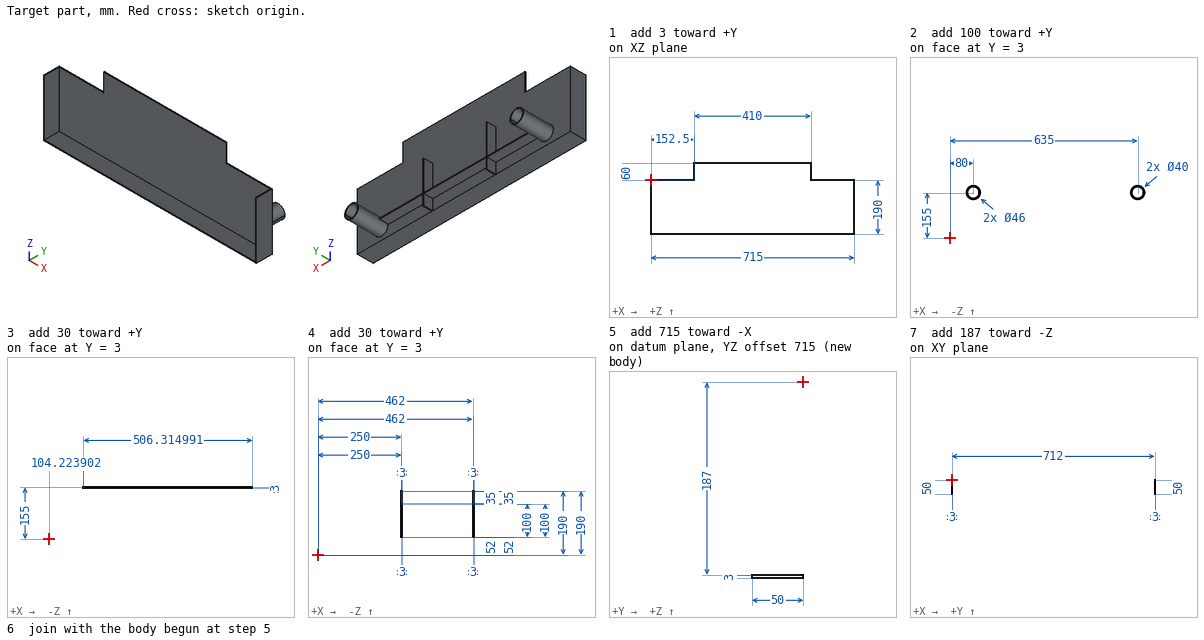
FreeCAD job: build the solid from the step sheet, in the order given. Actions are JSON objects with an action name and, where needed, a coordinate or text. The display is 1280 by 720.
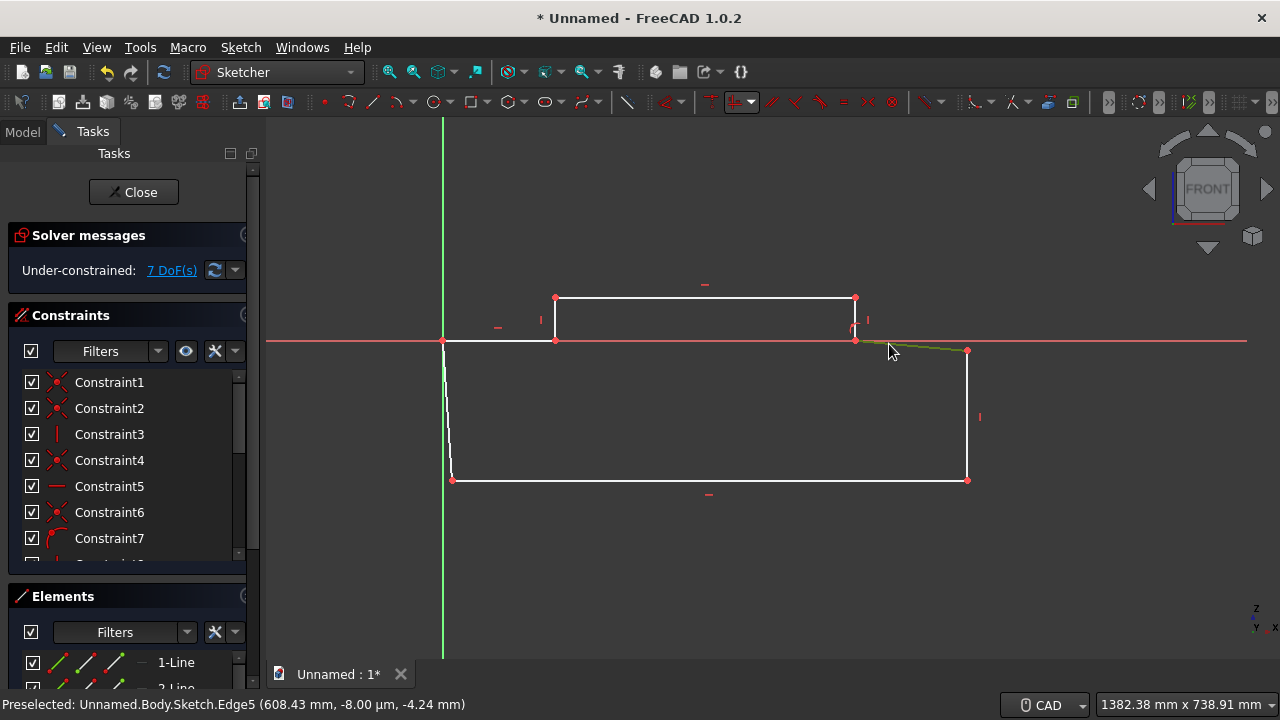
{"action": "key", "text": "h"}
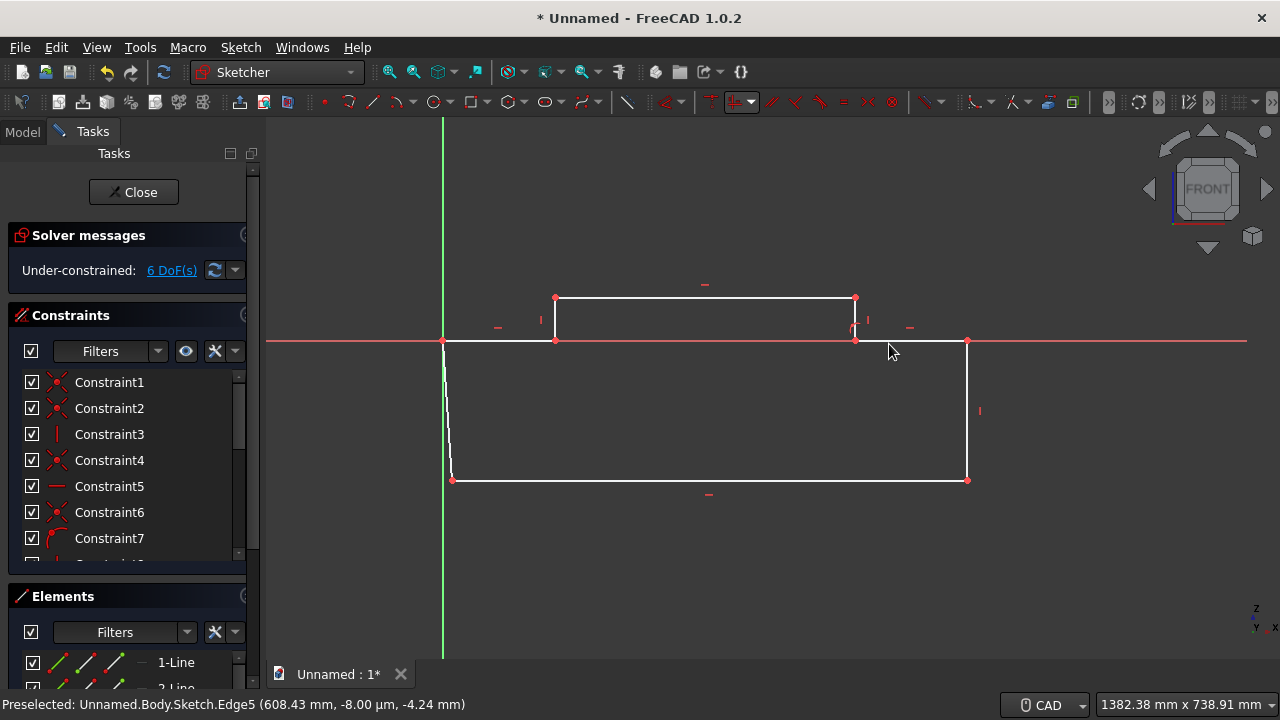
{"action": "left_click", "coordinate": [446, 383]}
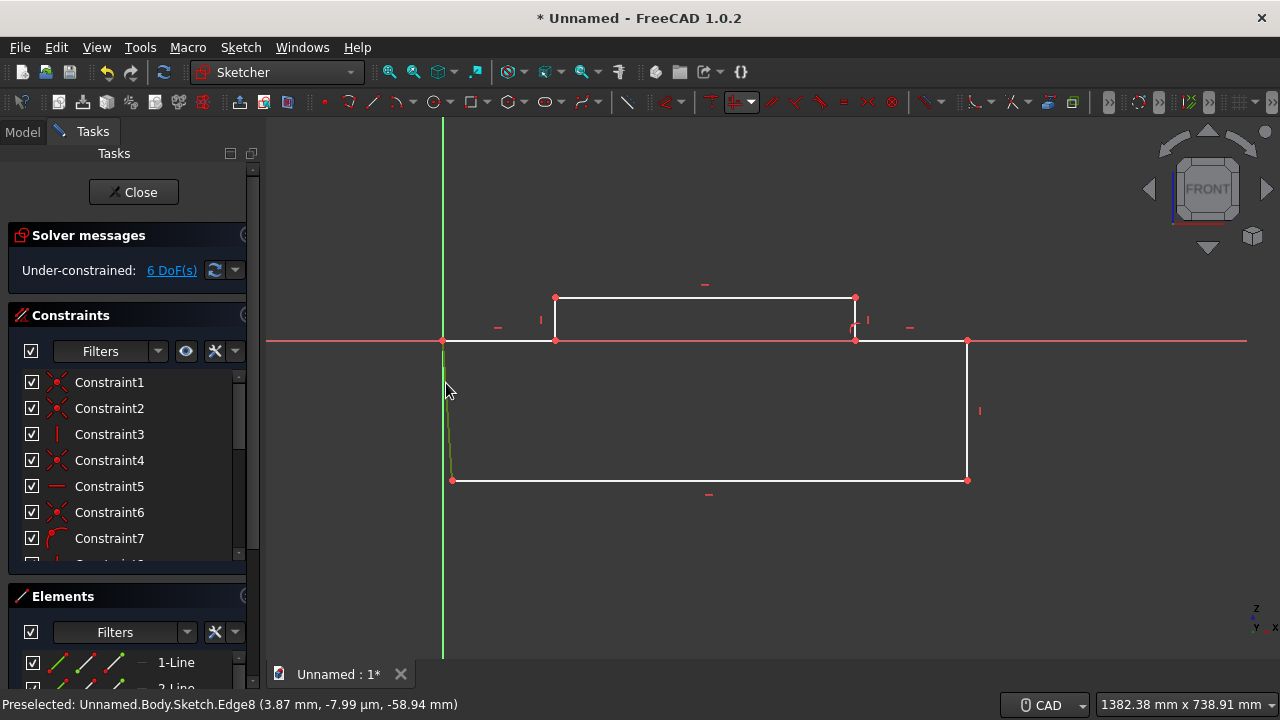
{"action": "key", "text": "v"}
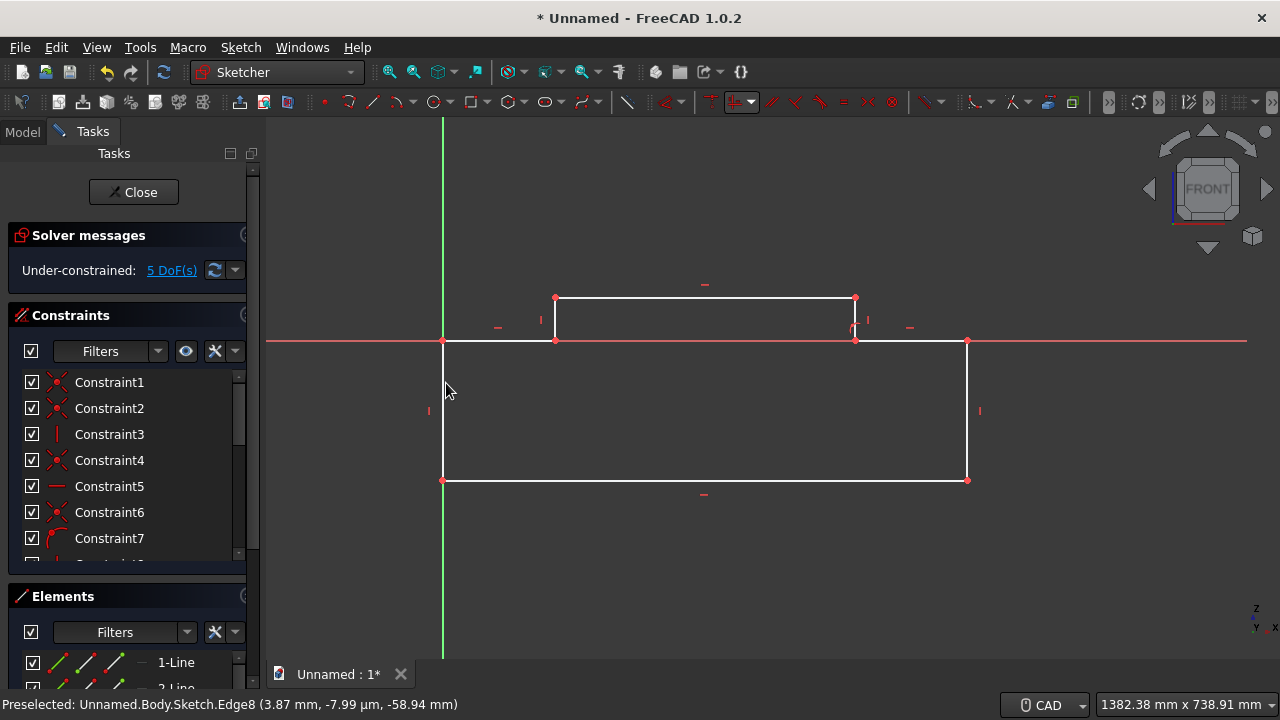
{"action": "key", "text": "d"}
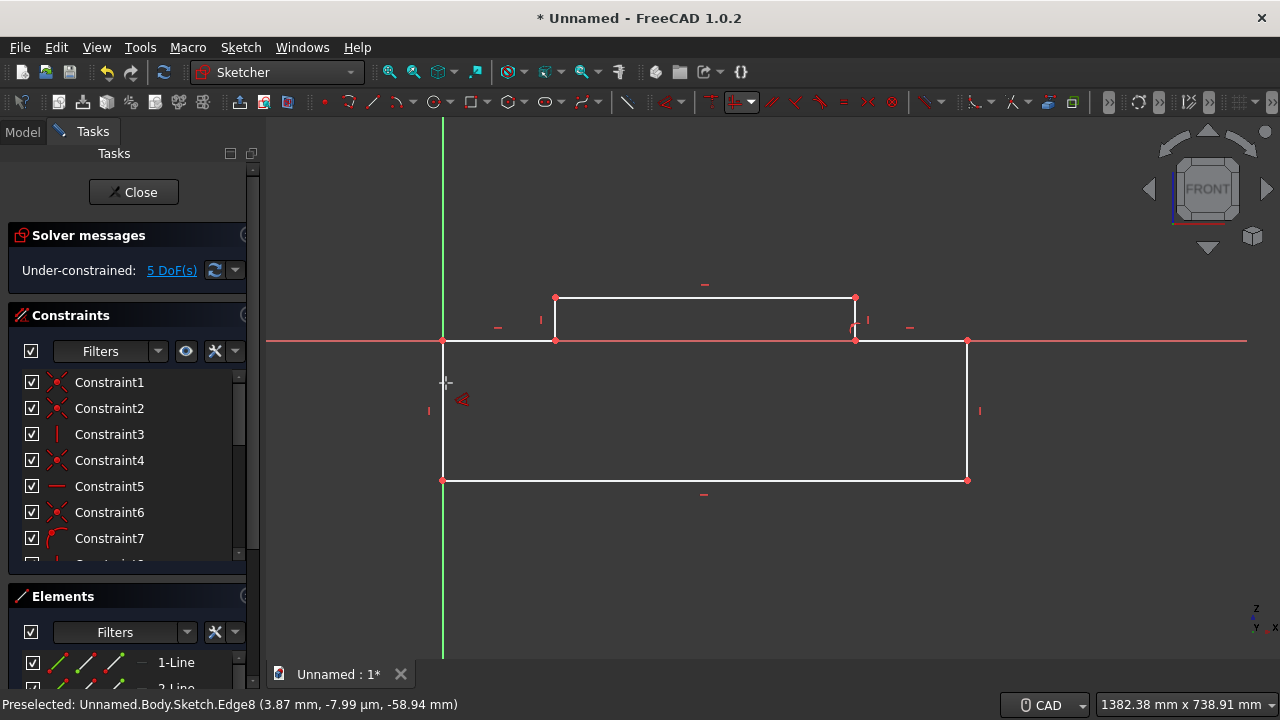
{"action": "left_click", "coordinate": [555, 328]}
{"action": "left_click", "coordinate": [521, 319]}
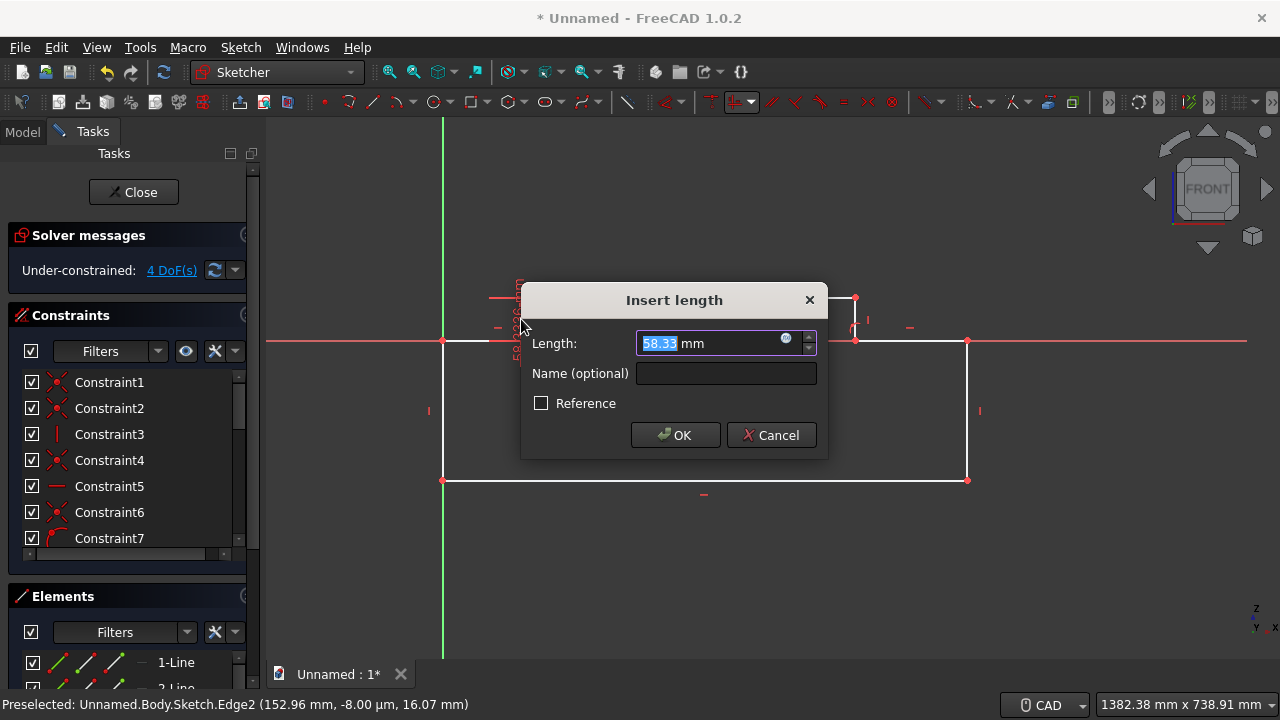
{"action": "type", "text": "60"}
{"action": "key", "text": "Return"}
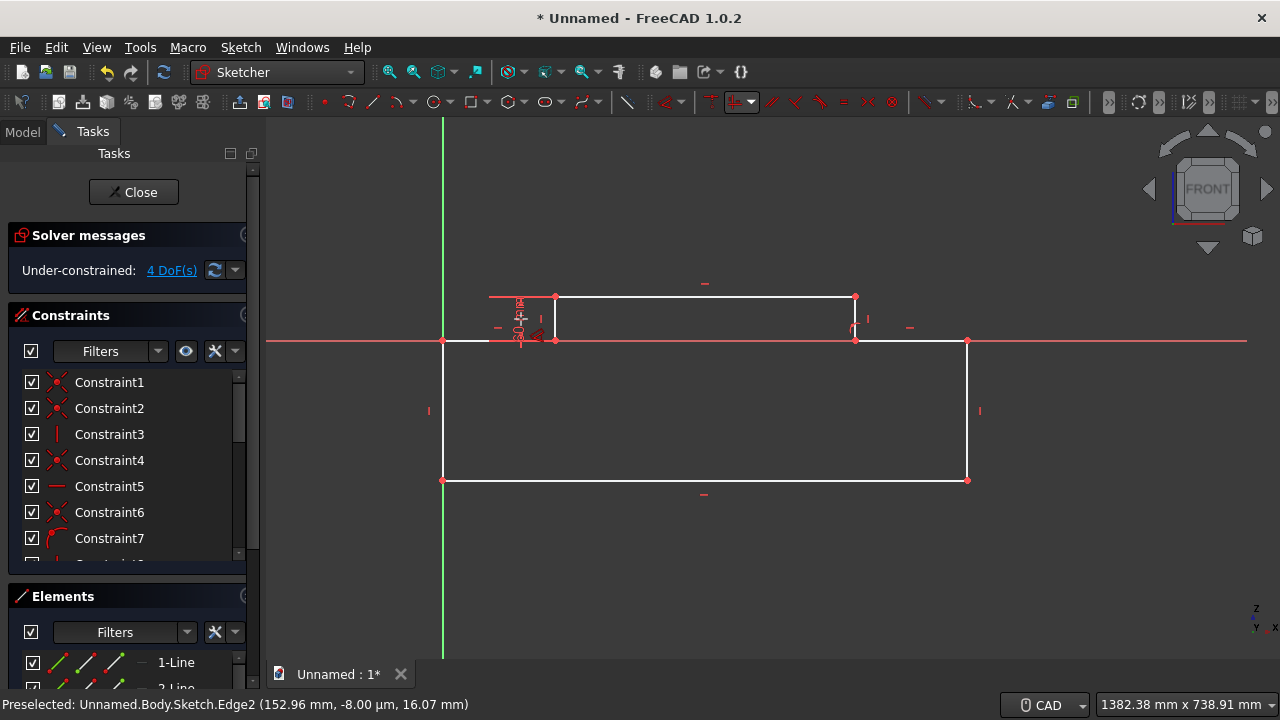
{"action": "left_click", "coordinate": [645, 297]}
{"action": "left_click", "coordinate": [705, 263]}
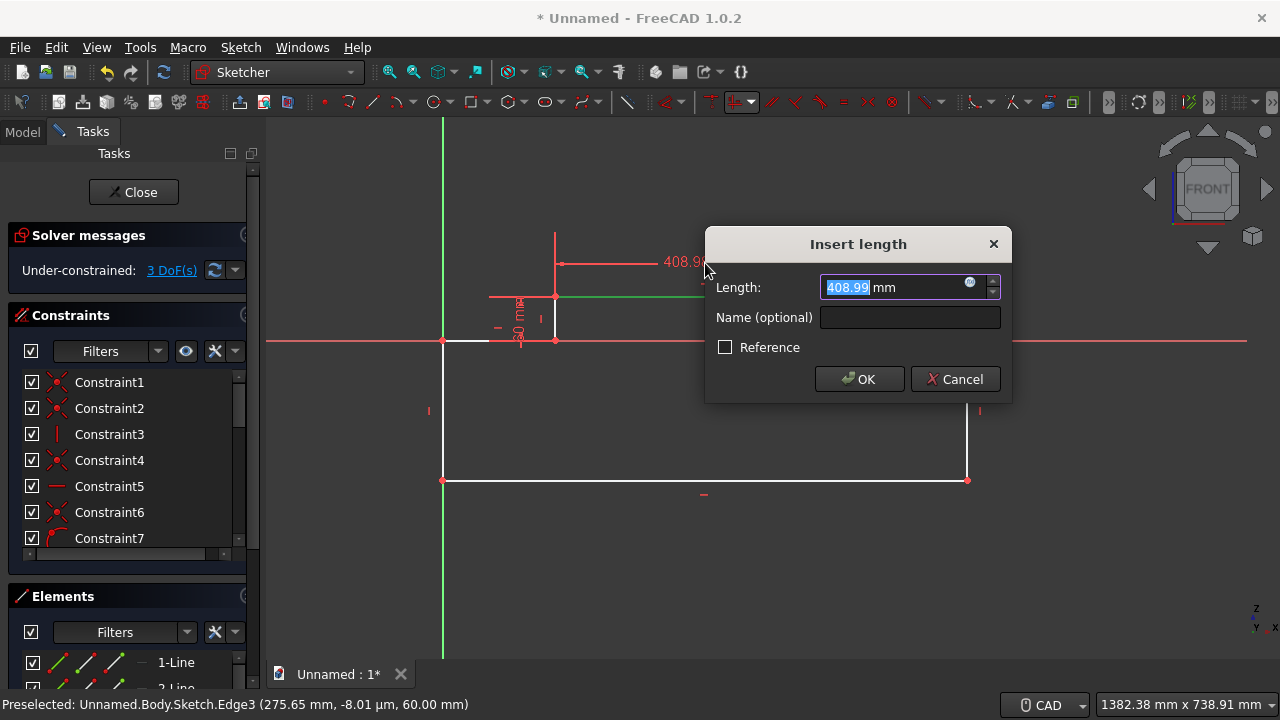
{"action": "type", "text": "410"}
{"action": "key", "text": "Return"}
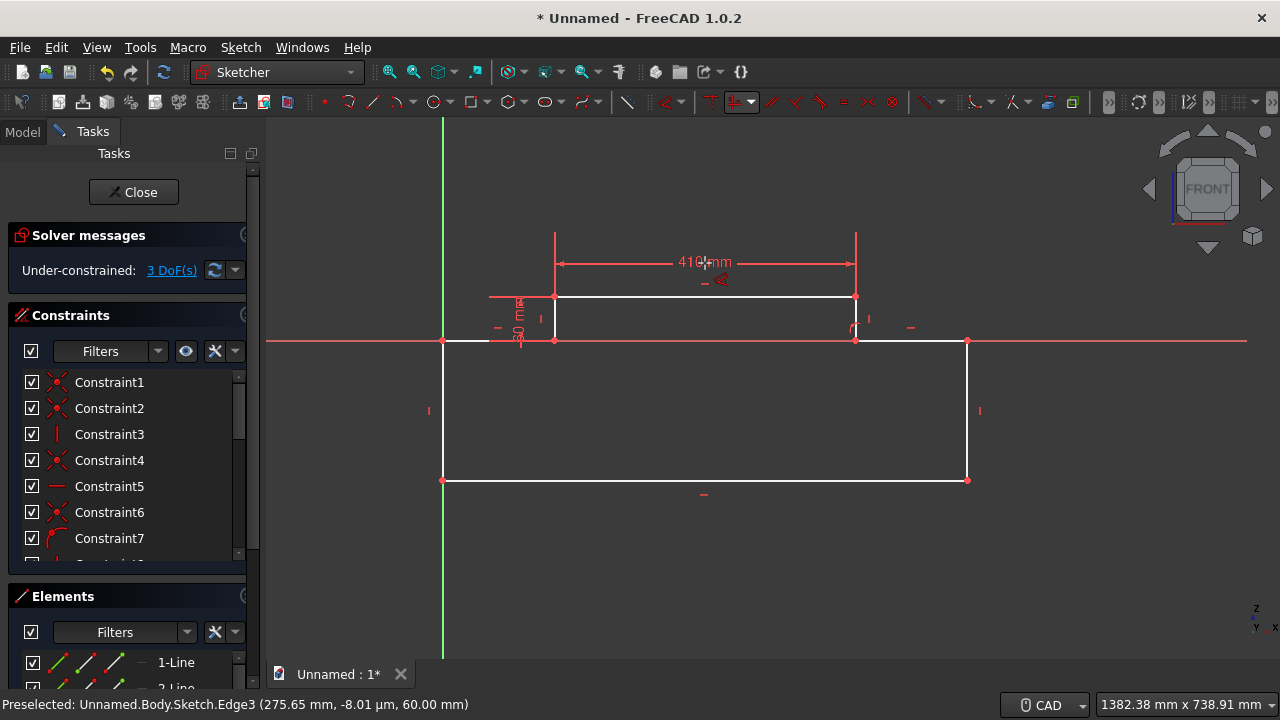
{"action": "left_click", "coordinate": [967, 383]}
{"action": "left_click", "coordinate": [1001, 411]}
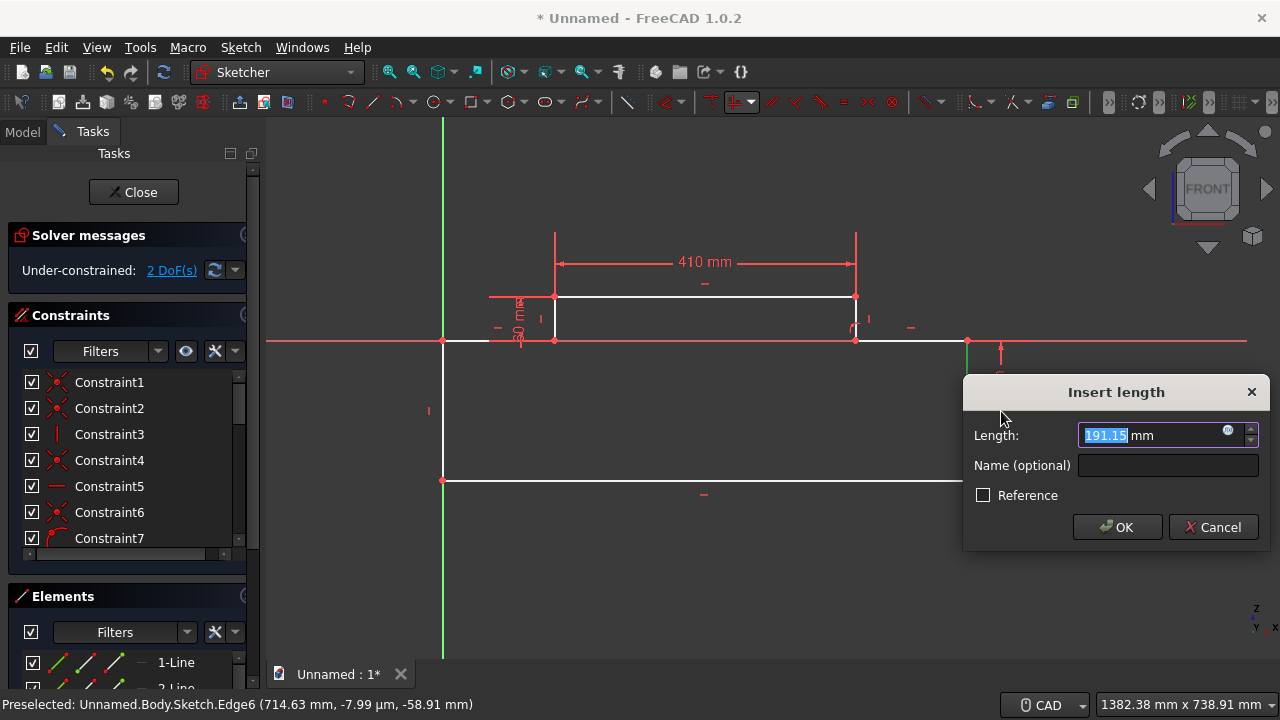
{"action": "type", "text": "190"}
{"action": "key", "text": "Return"}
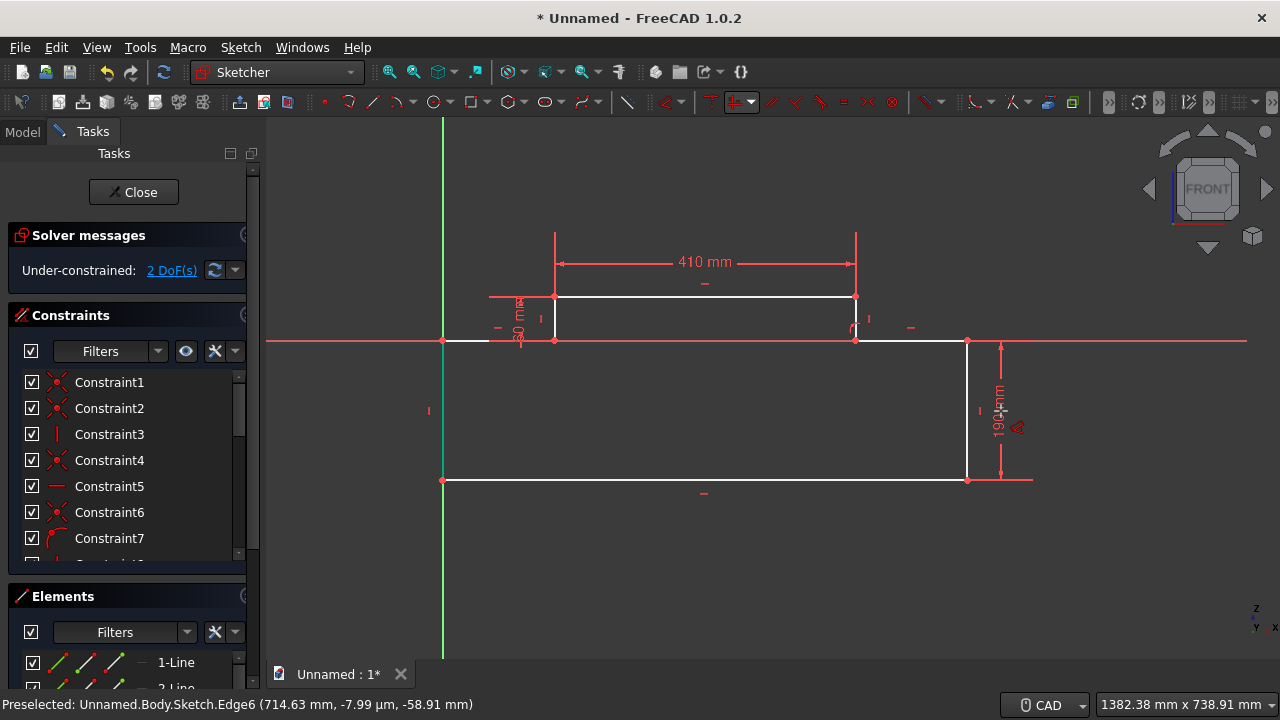
{"action": "left_click", "coordinate": [810, 480]}
{"action": "left_click", "coordinate": [705, 514]}